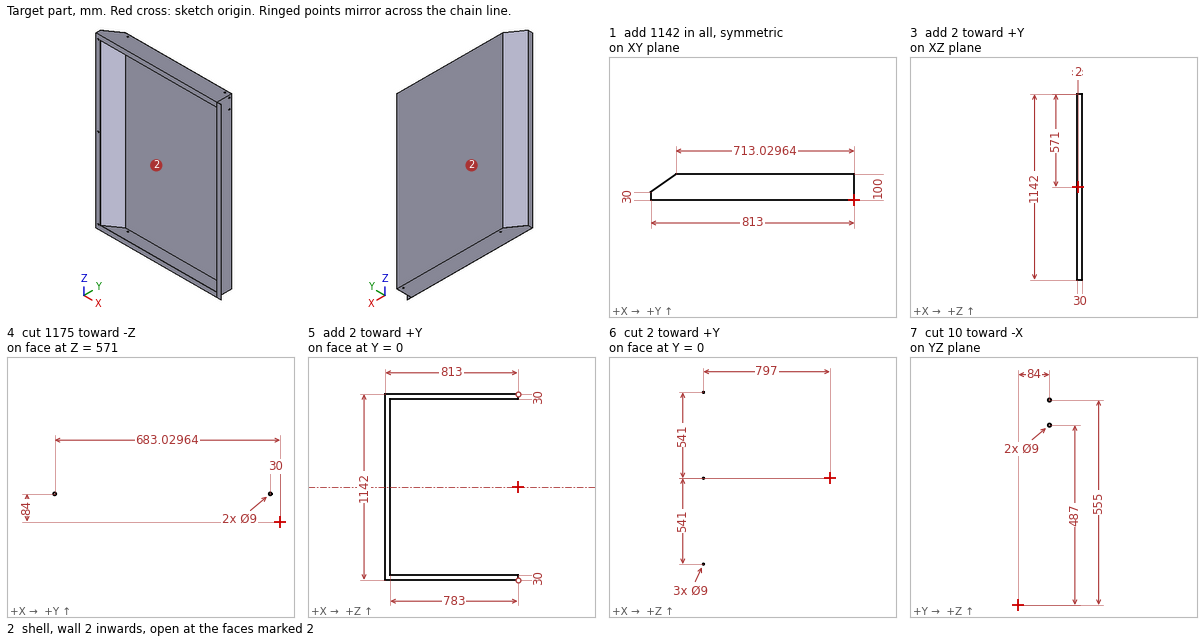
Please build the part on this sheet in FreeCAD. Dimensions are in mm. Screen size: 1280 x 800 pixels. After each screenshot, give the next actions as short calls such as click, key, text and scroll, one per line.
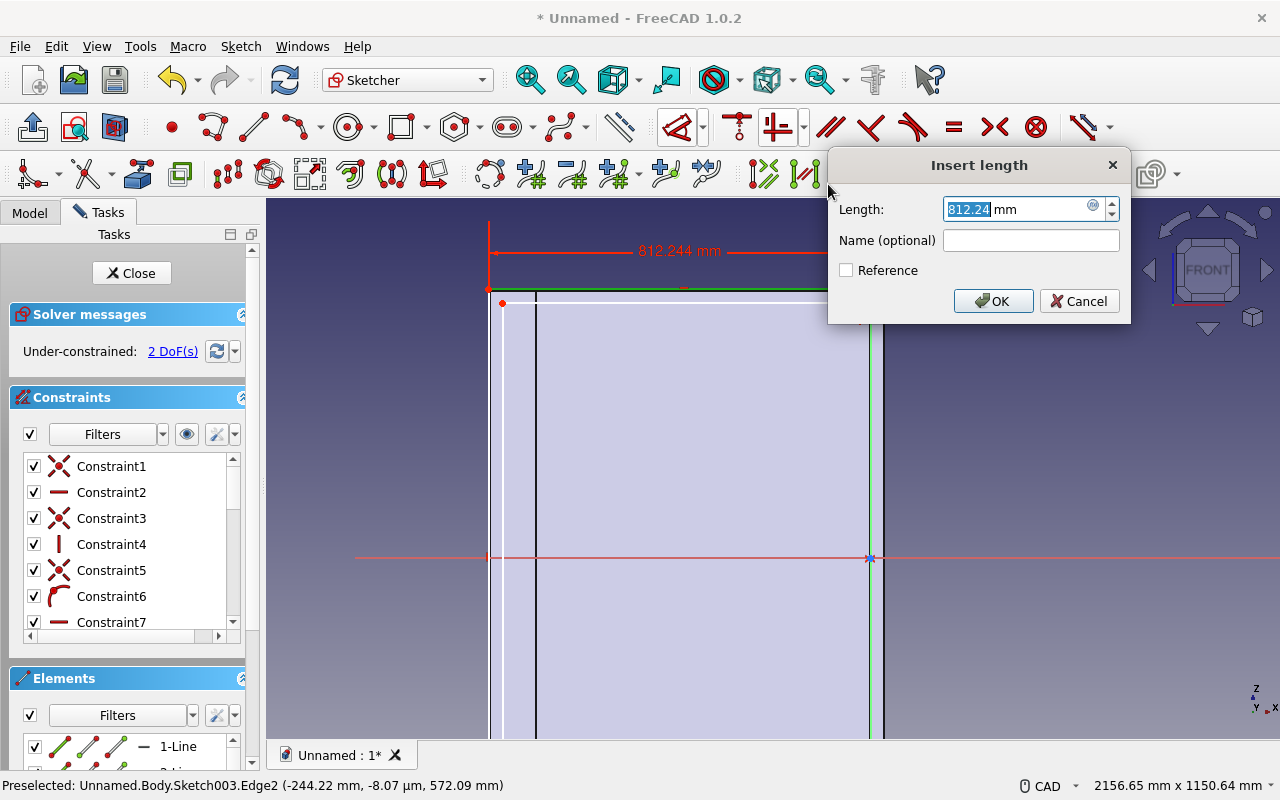
text(813)
key(Return)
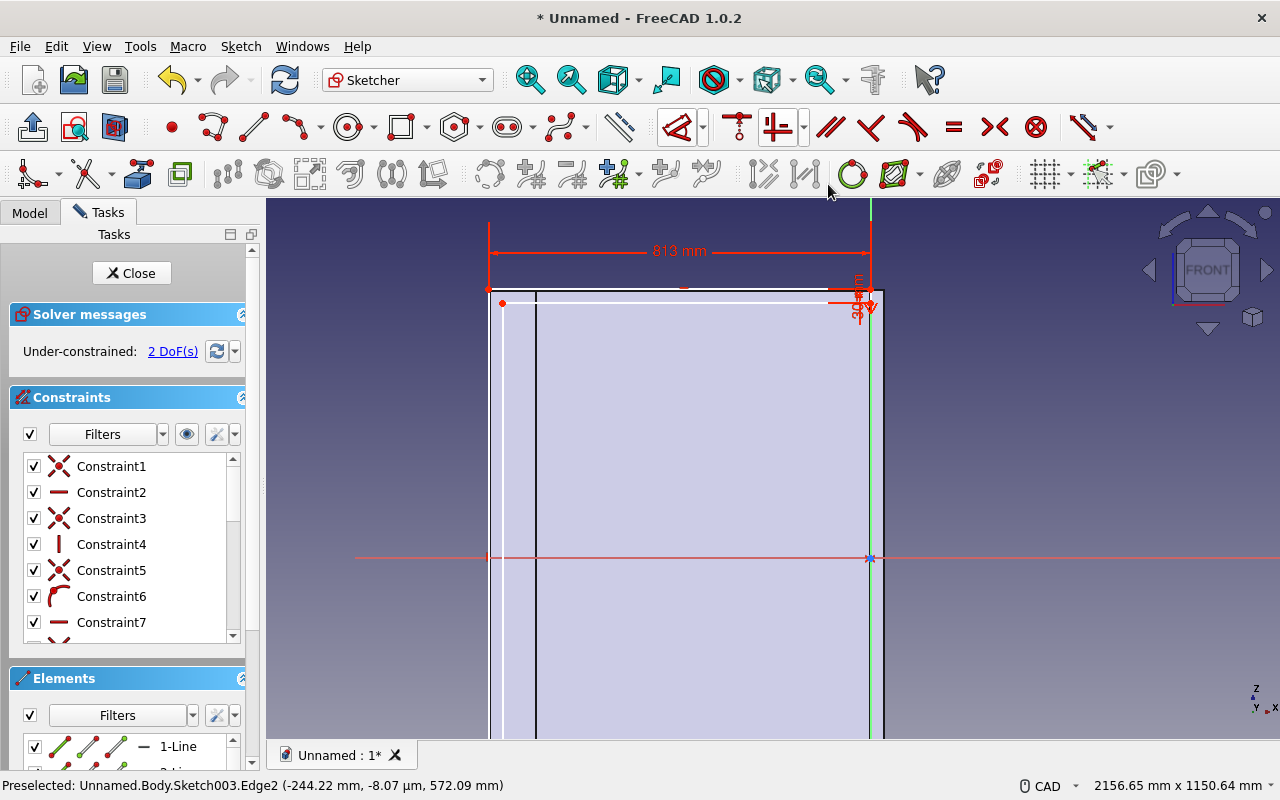
scroll(755, 286, down, 2)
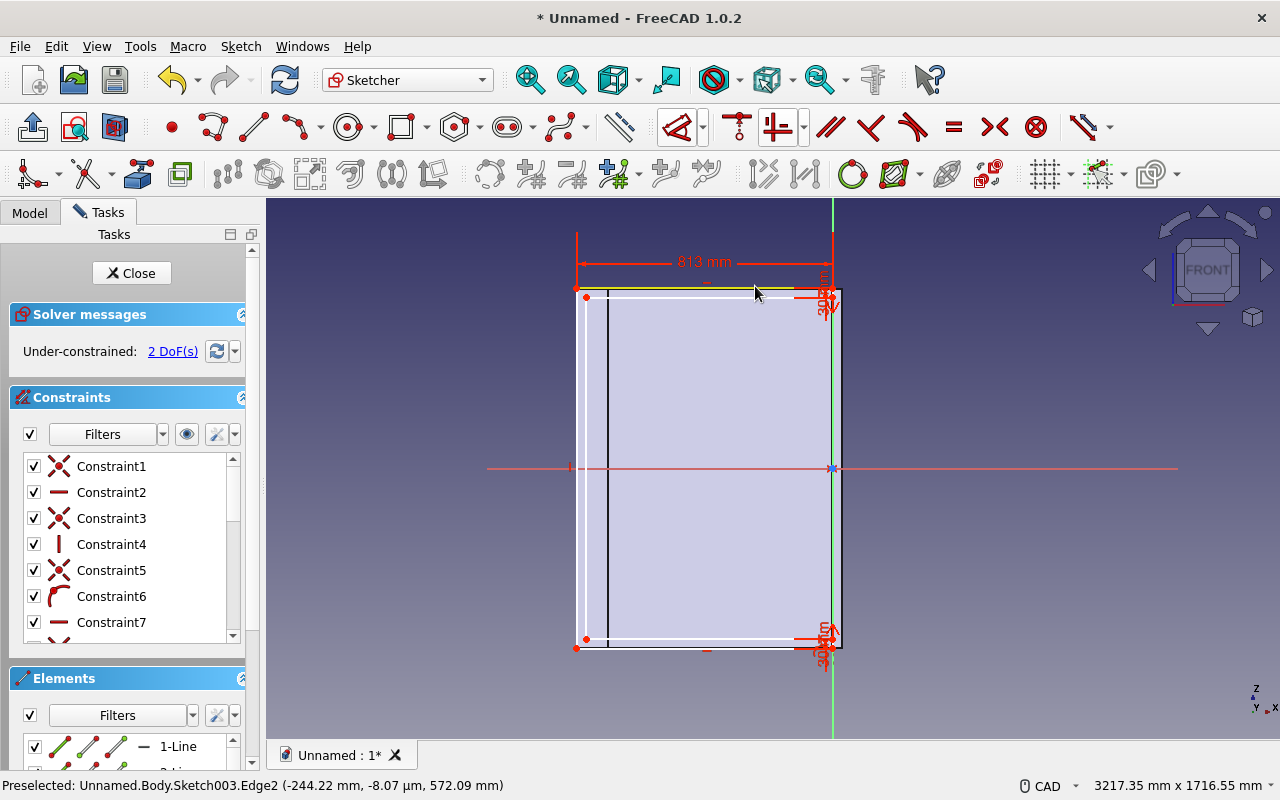
scroll(759, 639, up, 2)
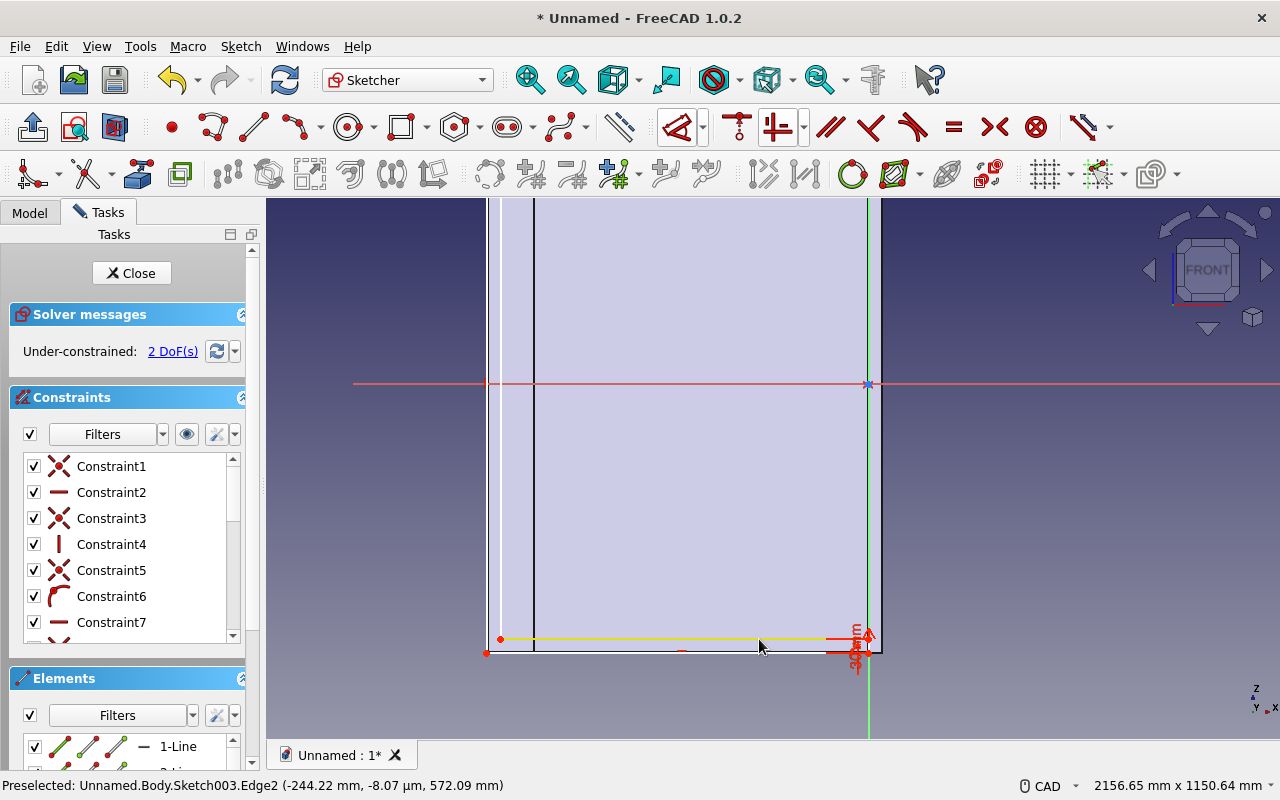
click(758, 639)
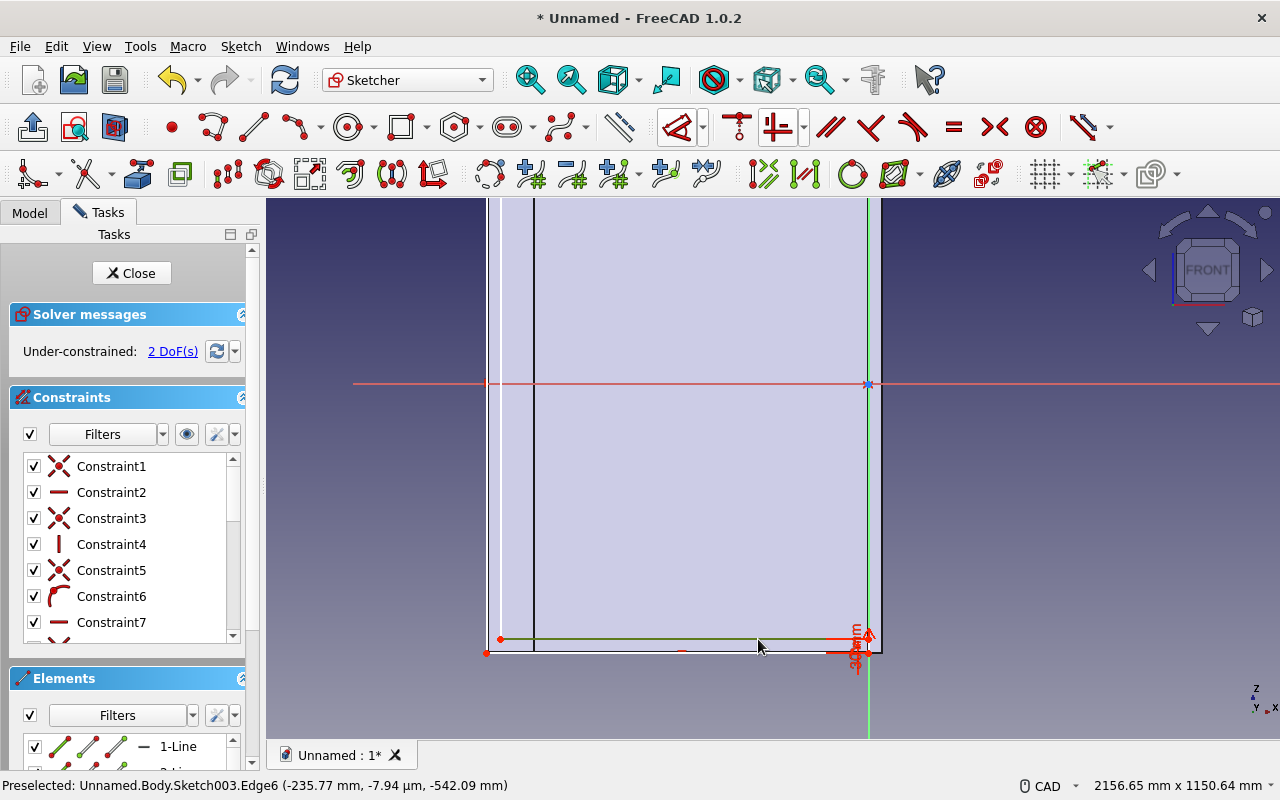
click(702, 128)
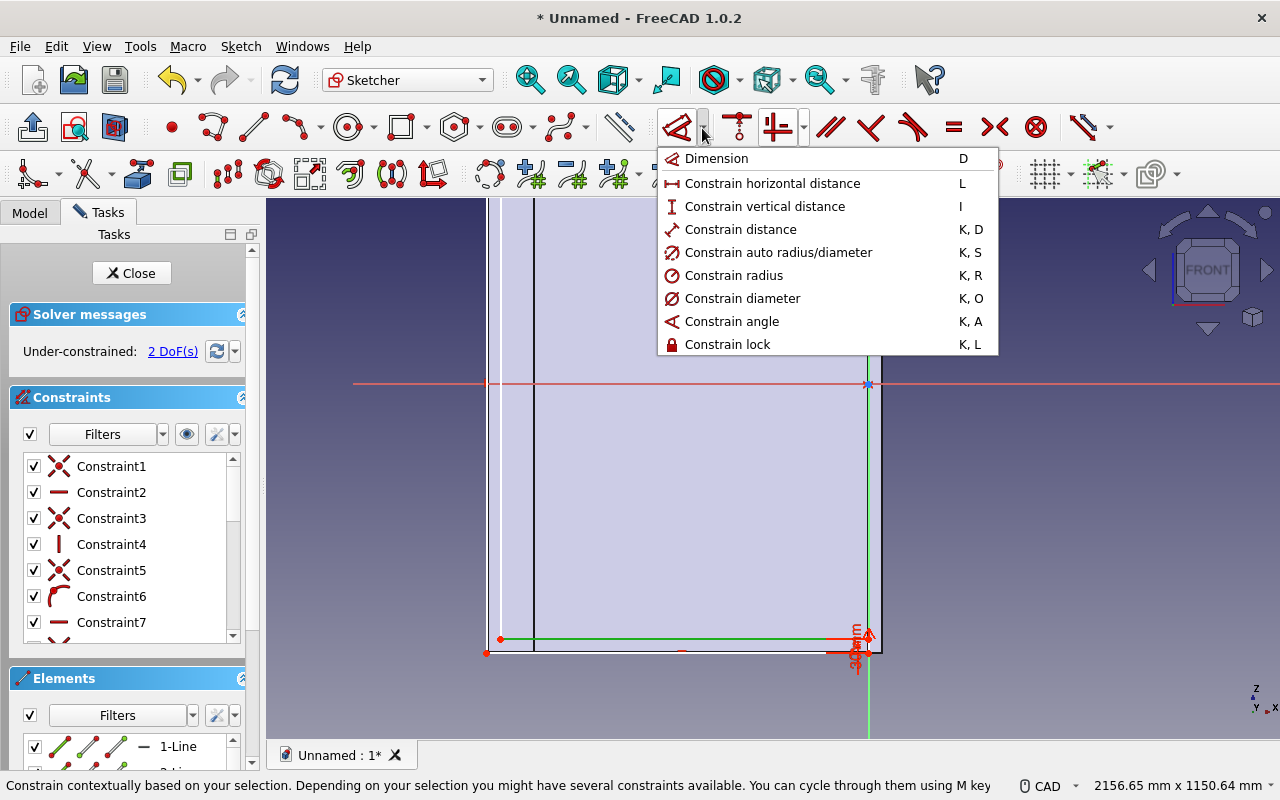
click(828, 184)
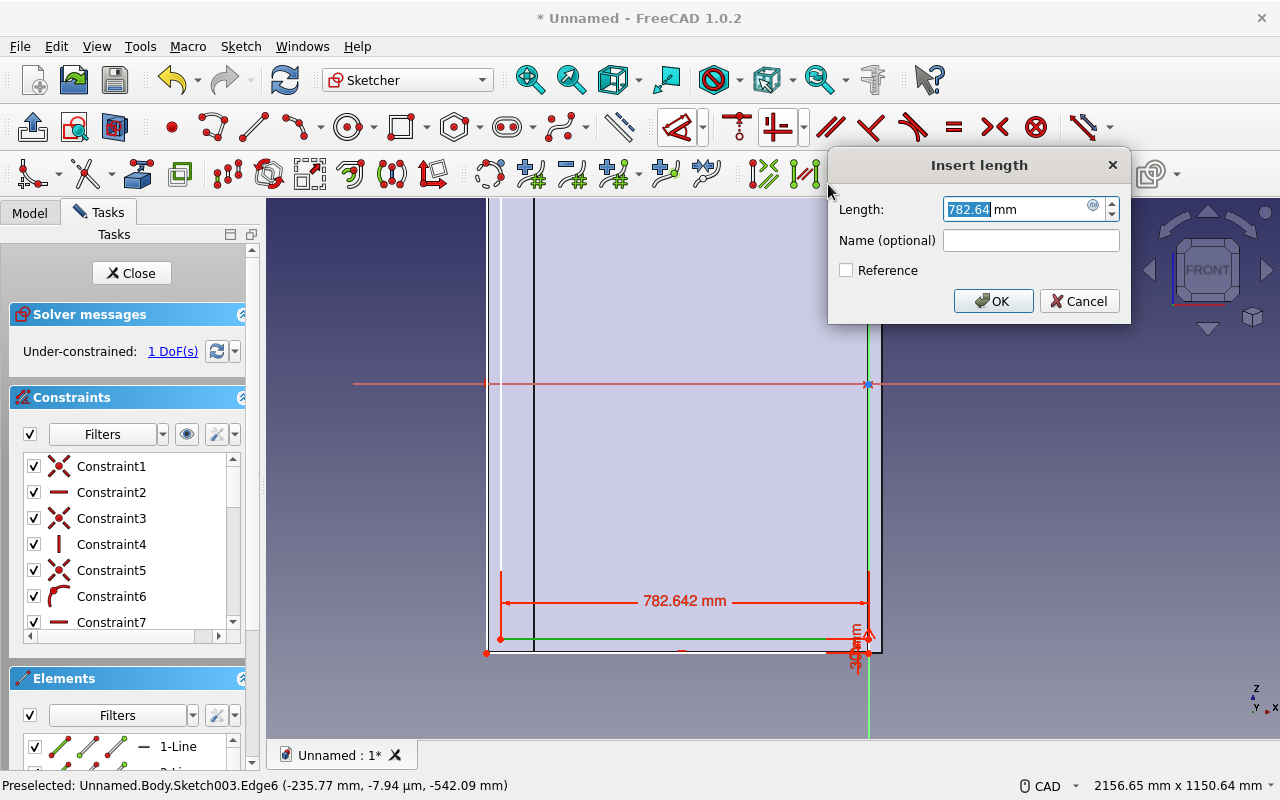
text(783)
key(Return)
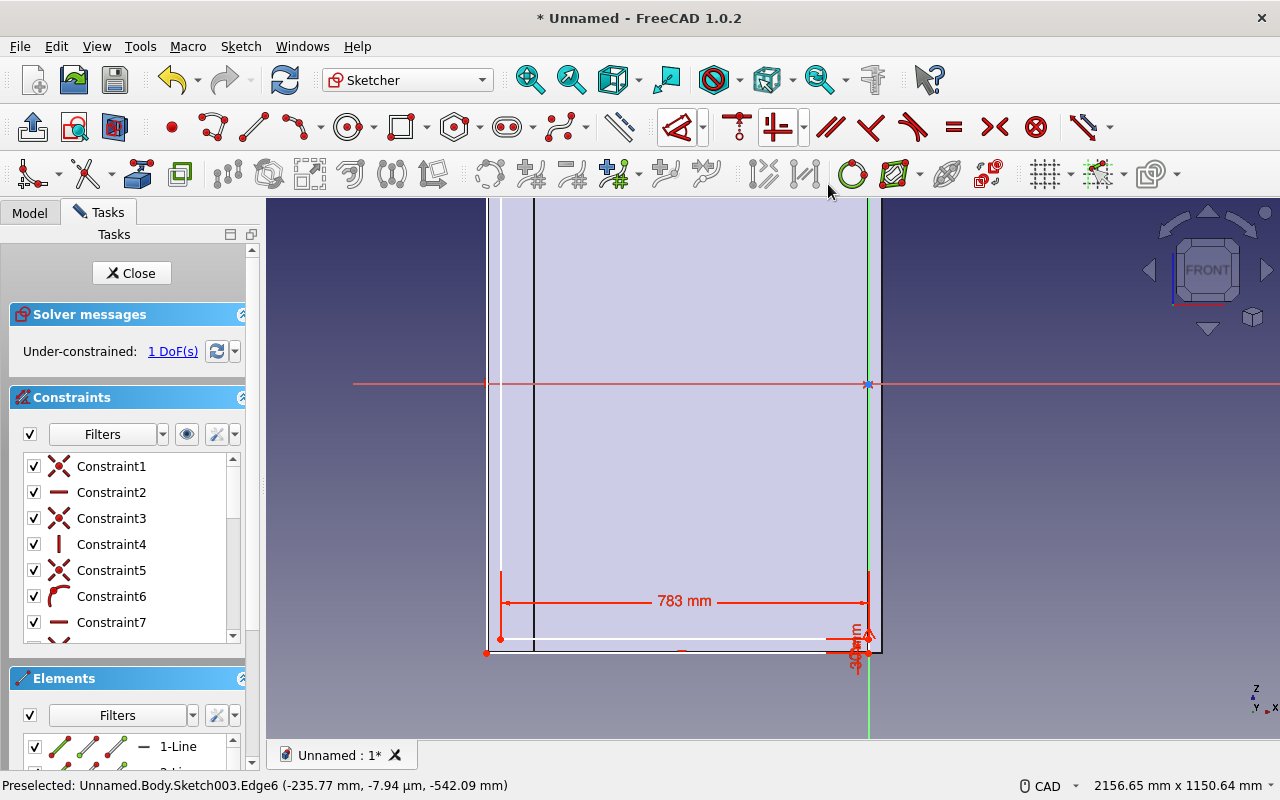
click(487, 277)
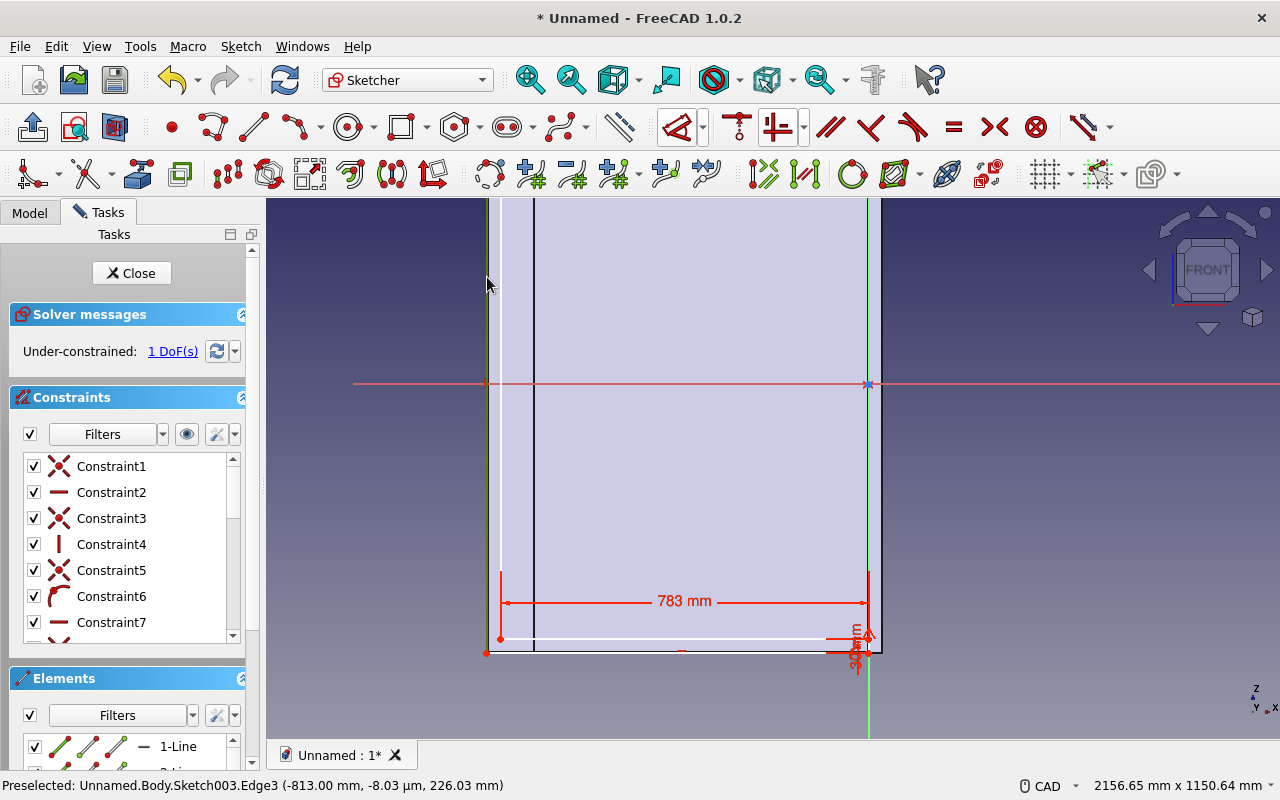
key(i)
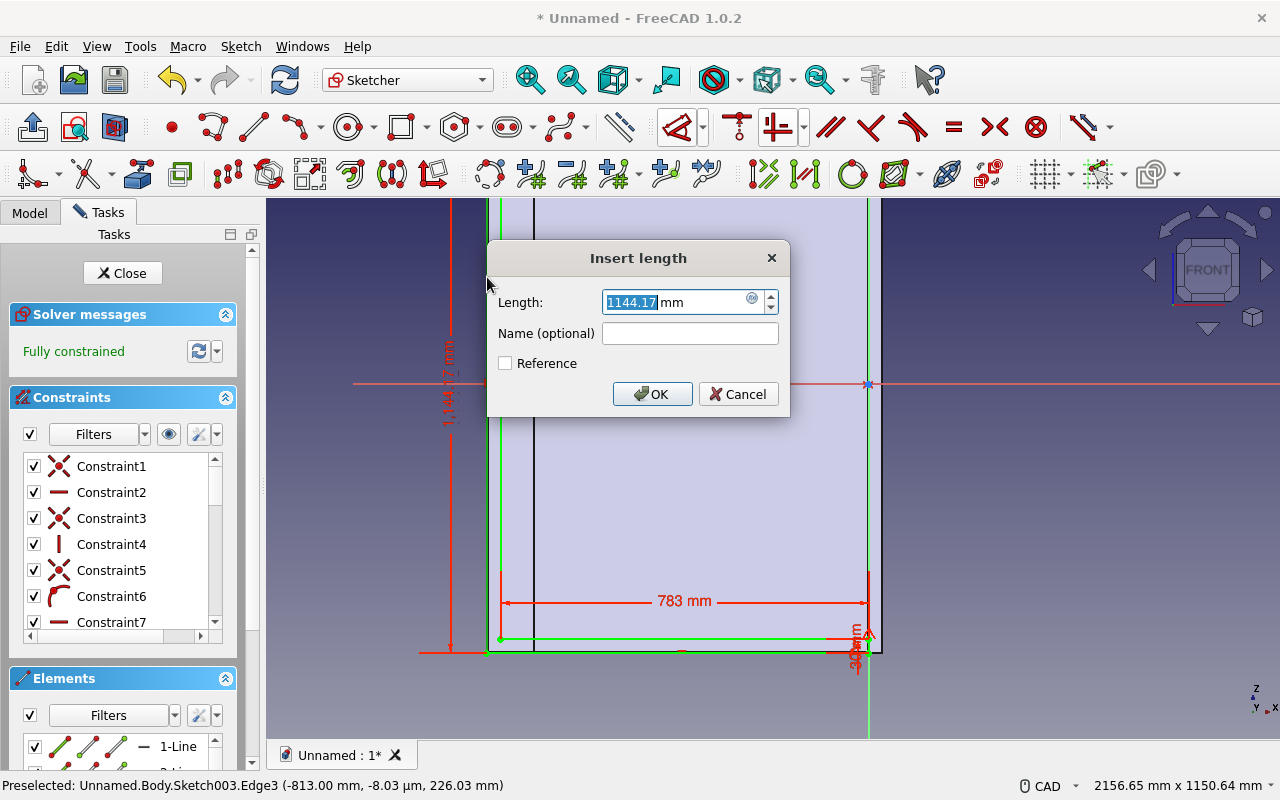
text(1142)
key(Return)